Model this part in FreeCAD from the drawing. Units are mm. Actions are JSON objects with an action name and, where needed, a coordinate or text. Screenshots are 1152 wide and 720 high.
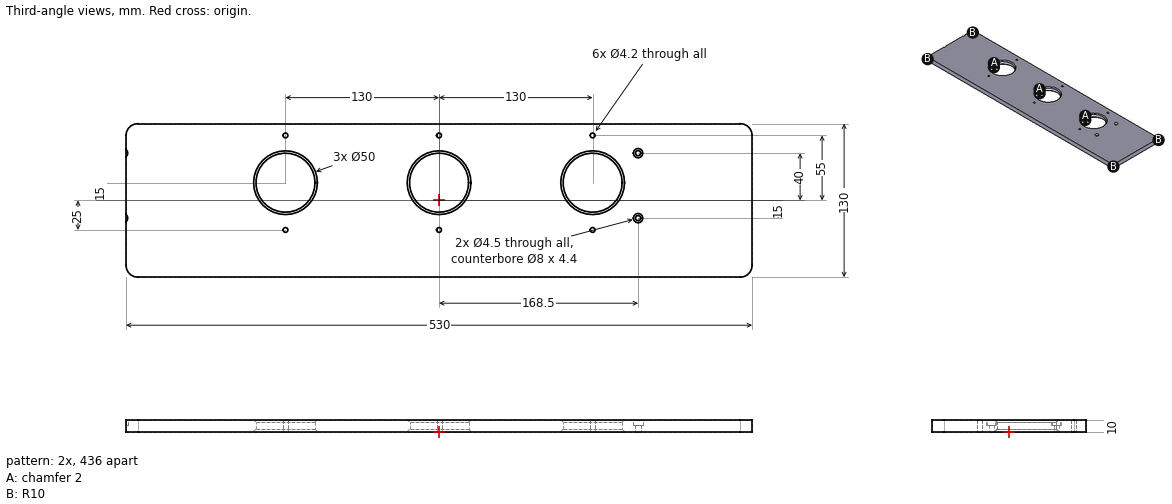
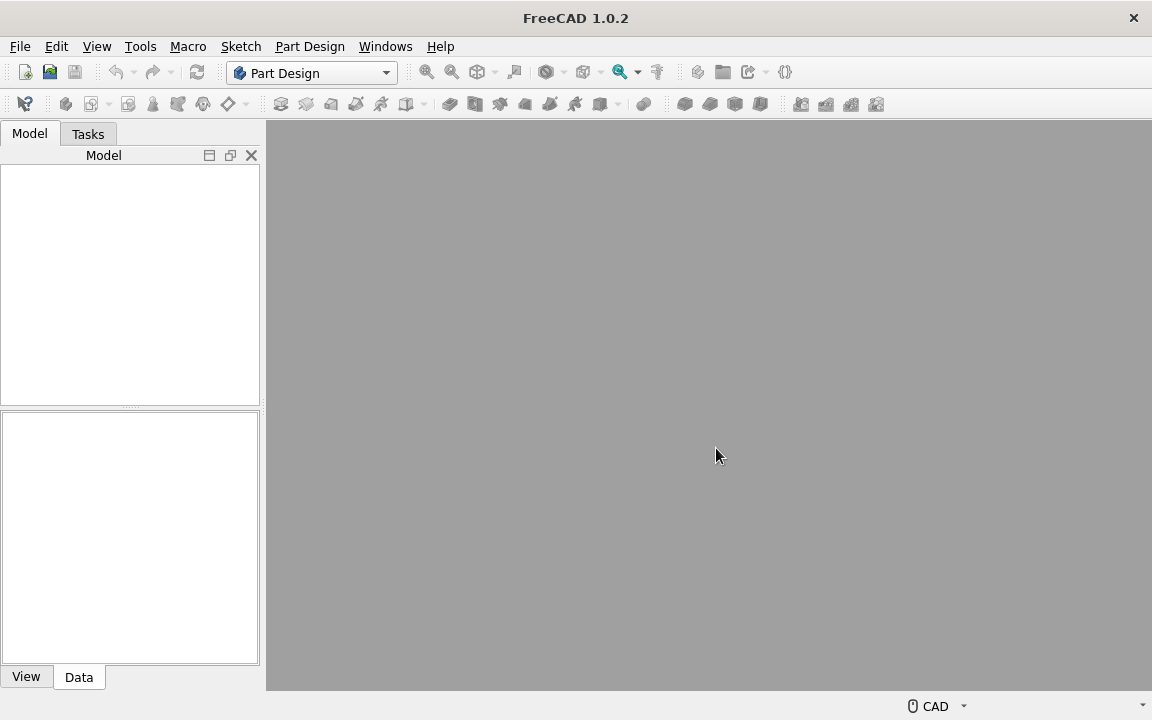
{"action": "left_click", "coordinate": [25, 72]}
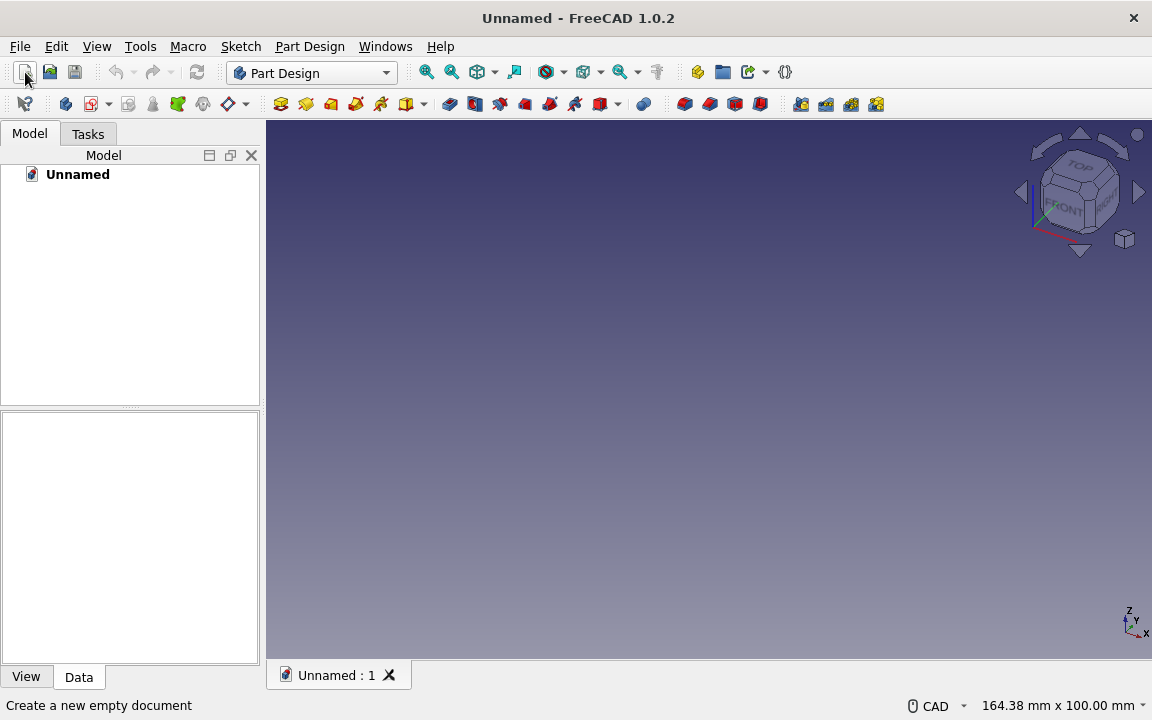
{"action": "left_click", "coordinate": [90, 104]}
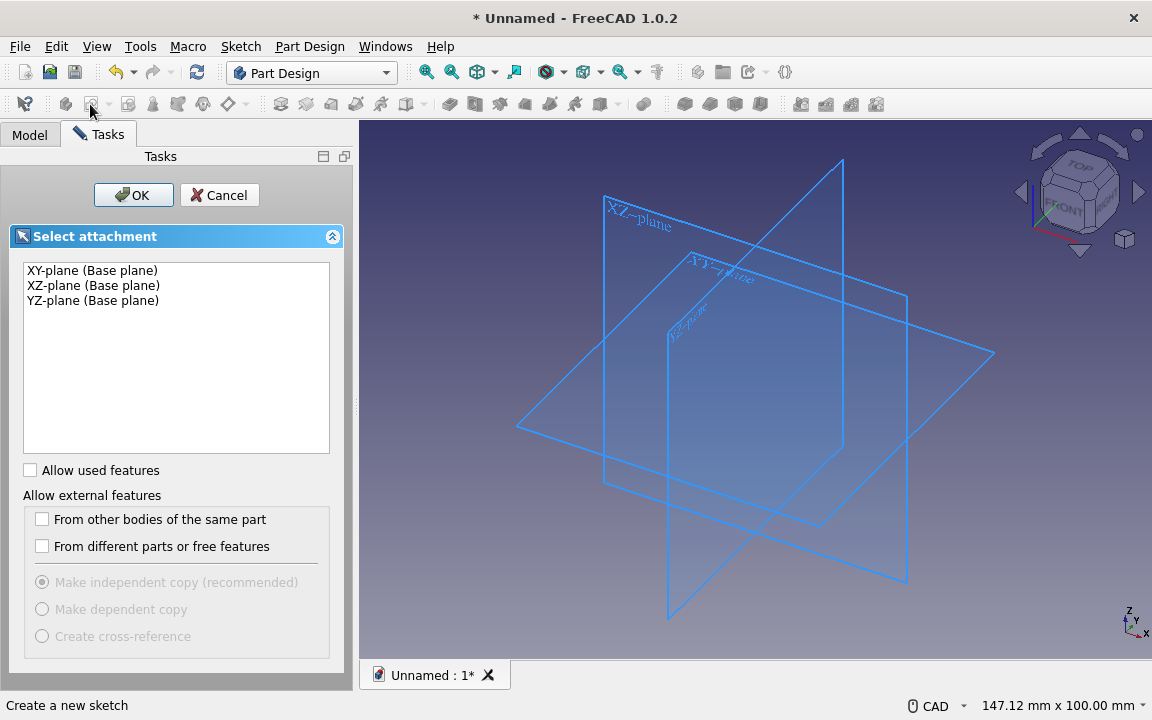
{"action": "left_click", "coordinate": [84, 270]}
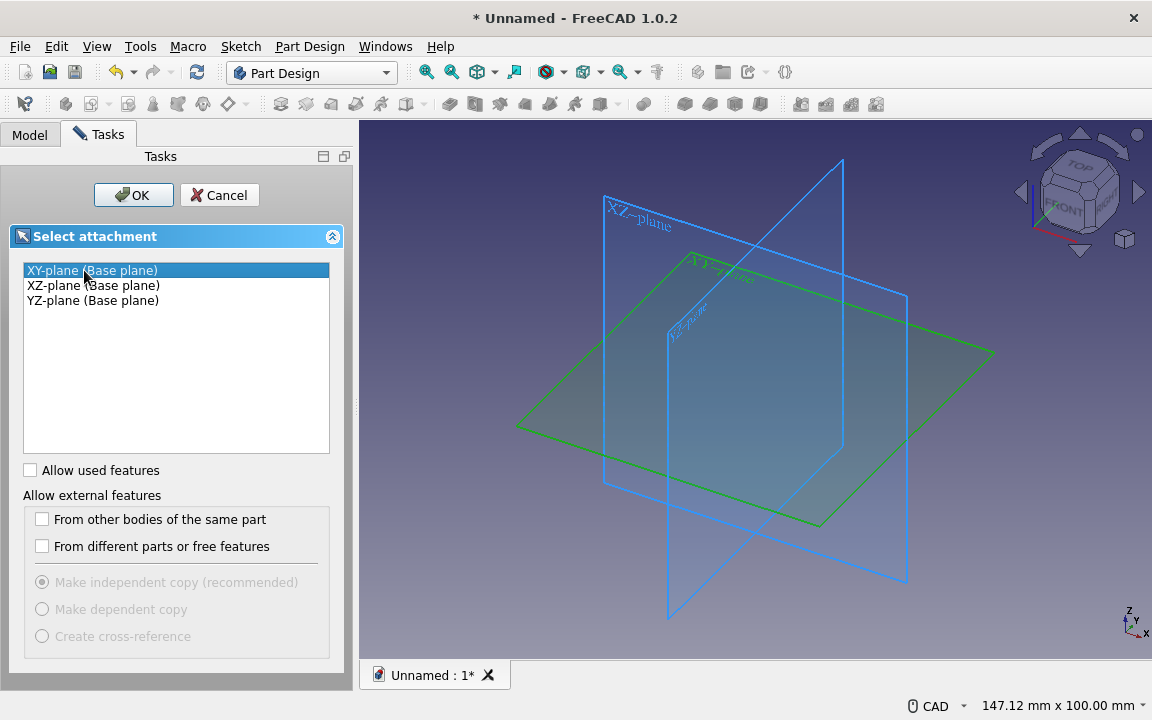
{"action": "left_click", "coordinate": [134, 195]}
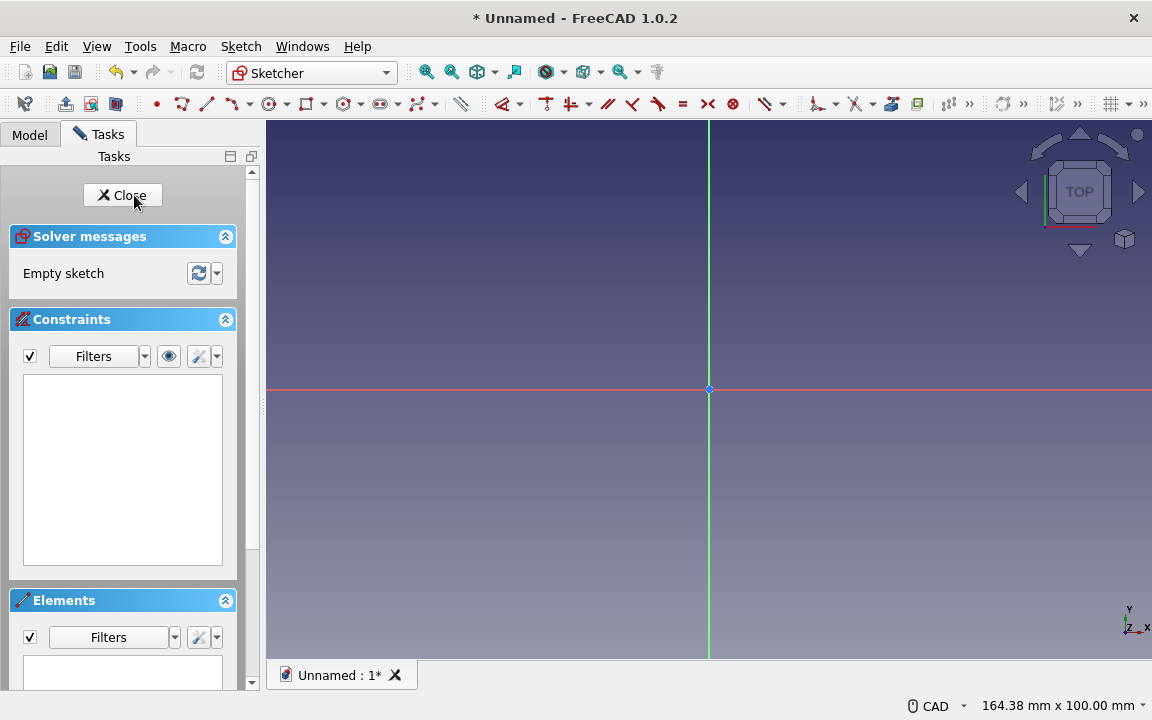
{"action": "scroll", "coordinate": [627, 390], "scroll_direction": "down", "scroll_amount": 9}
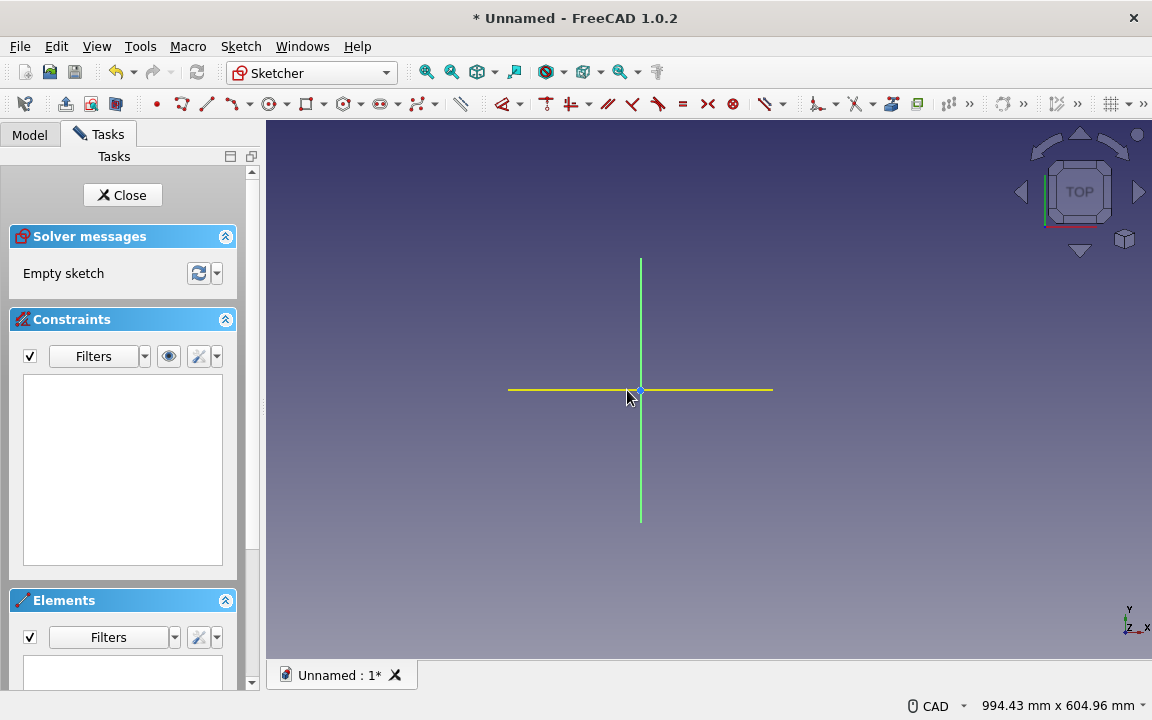
{"action": "left_click", "coordinate": [324, 104]}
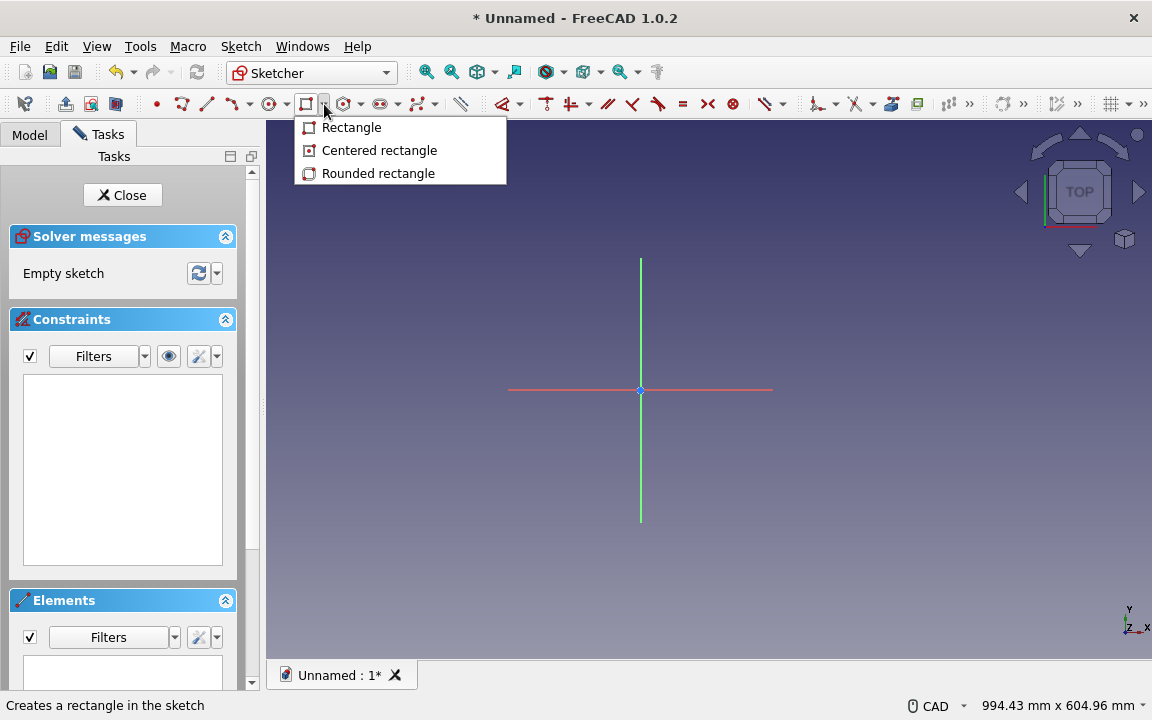
{"action": "left_click", "coordinate": [400, 150]}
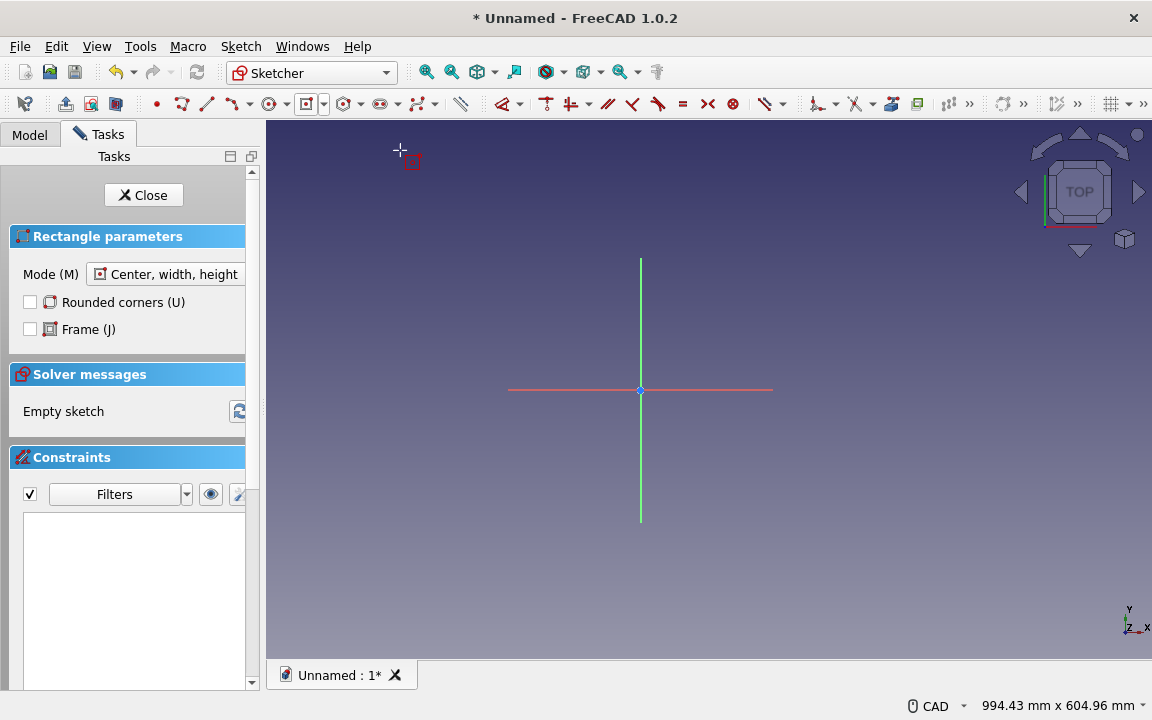
{"action": "left_click", "coordinate": [641, 390]}
{"action": "mouse_move", "coordinate": [877, 332]}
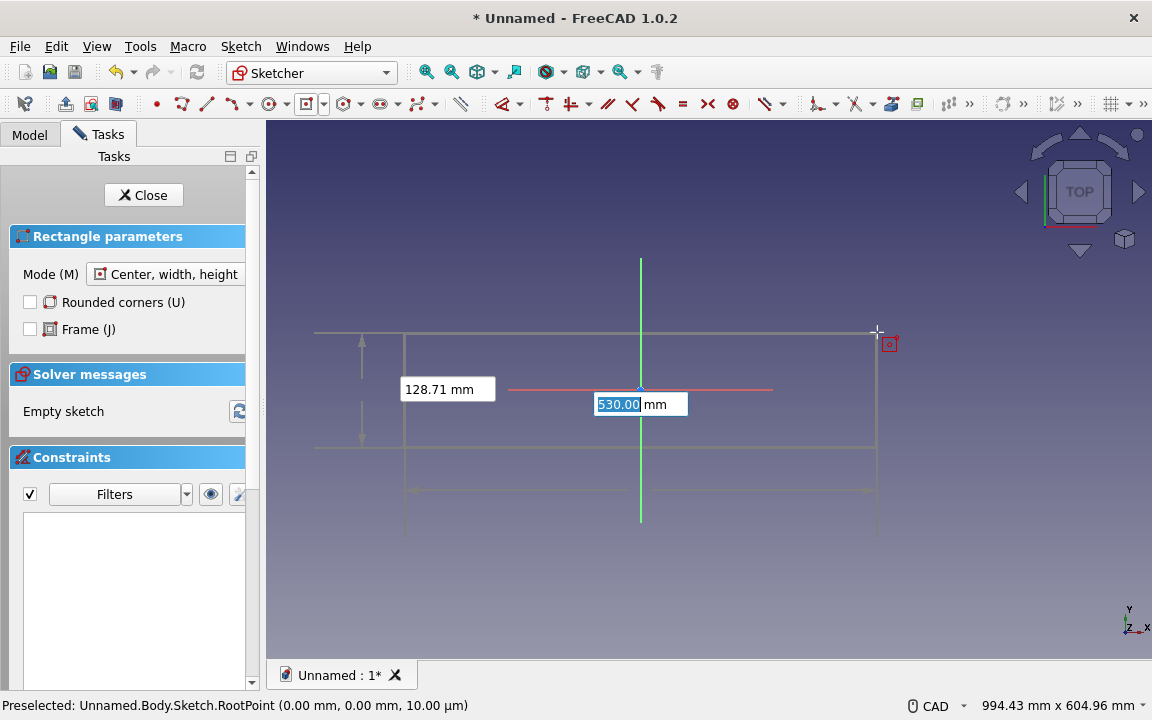
{"action": "type", "text": "530"}
{"action": "key", "text": "Tab"}
{"action": "type", "text": "130"}
{"action": "key", "text": "Return"}
{"action": "key", "text": "Escape"}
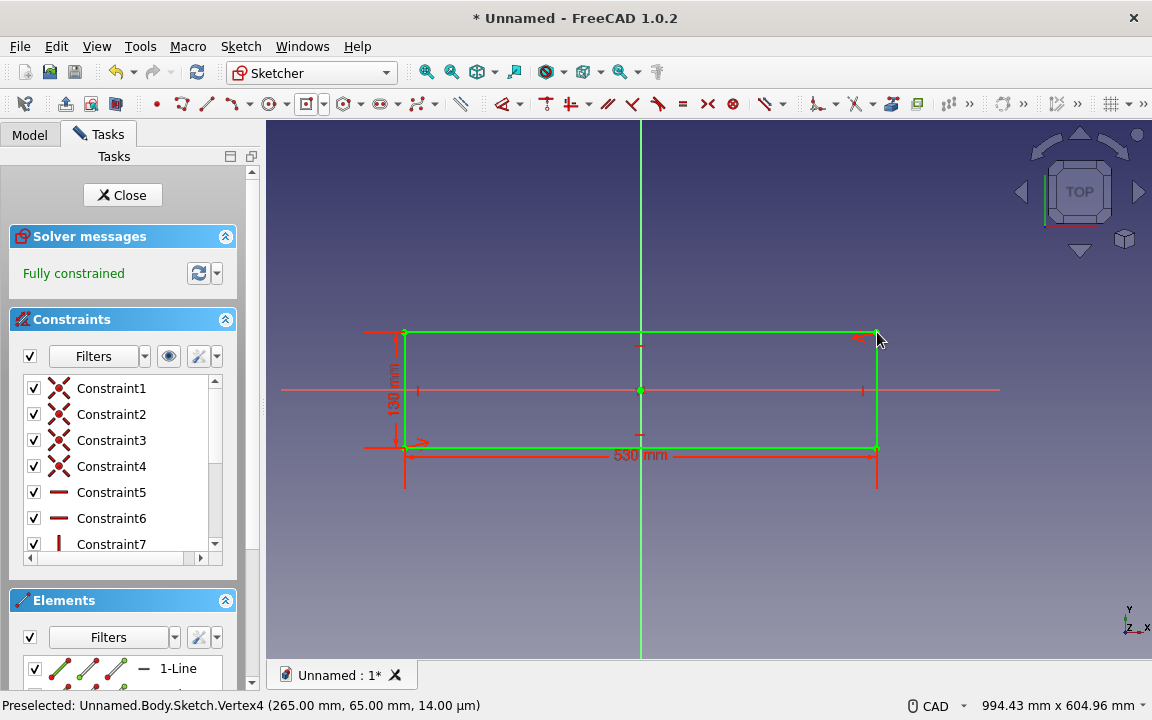
{"action": "left_click", "coordinate": [123, 195]}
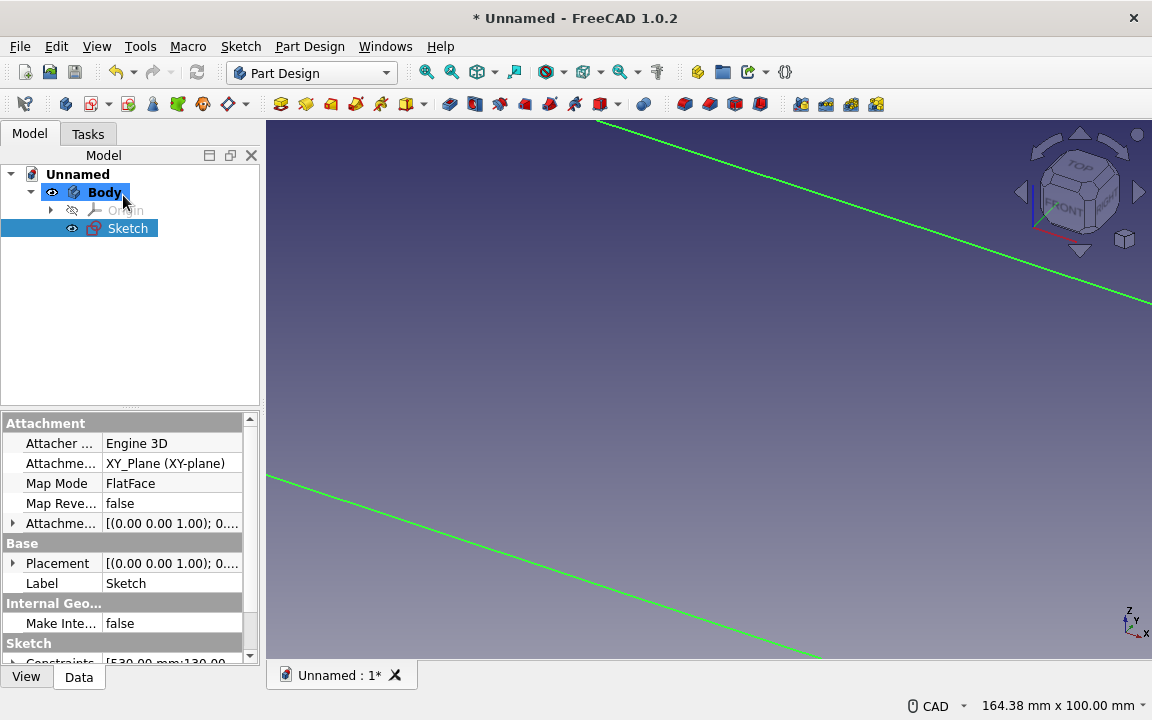
{"action": "left_click", "coordinate": [281, 104]}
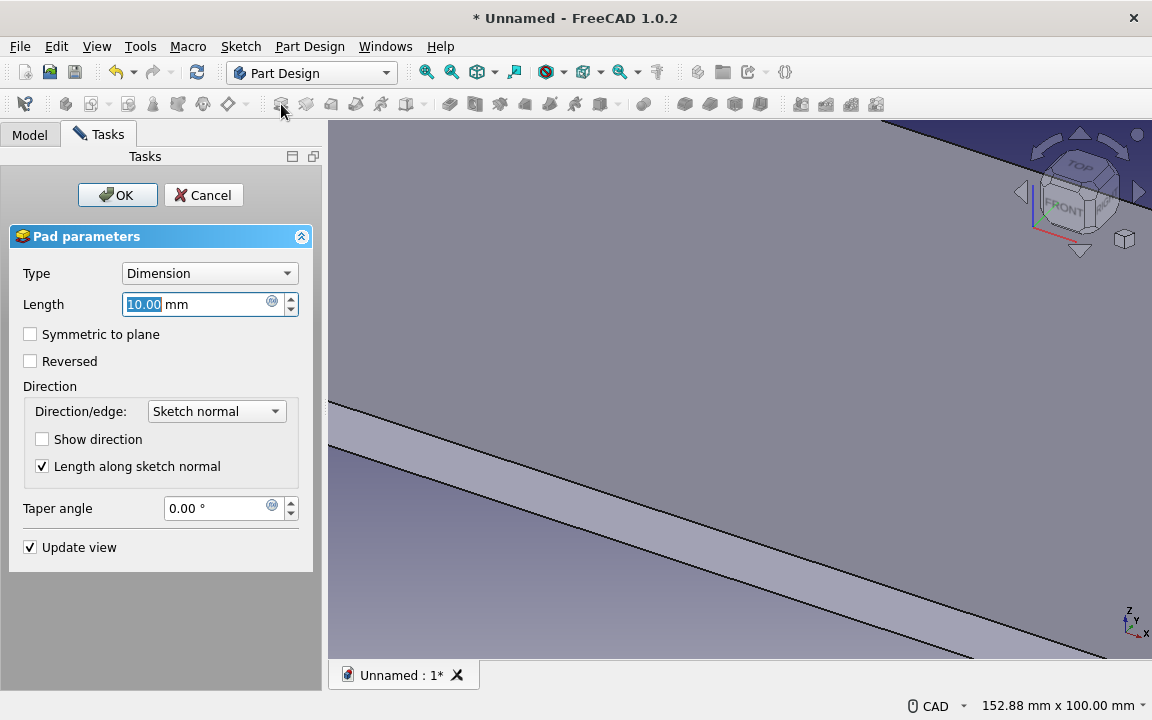
{"action": "type", "text": "10"}
{"action": "key", "text": "Tab"}